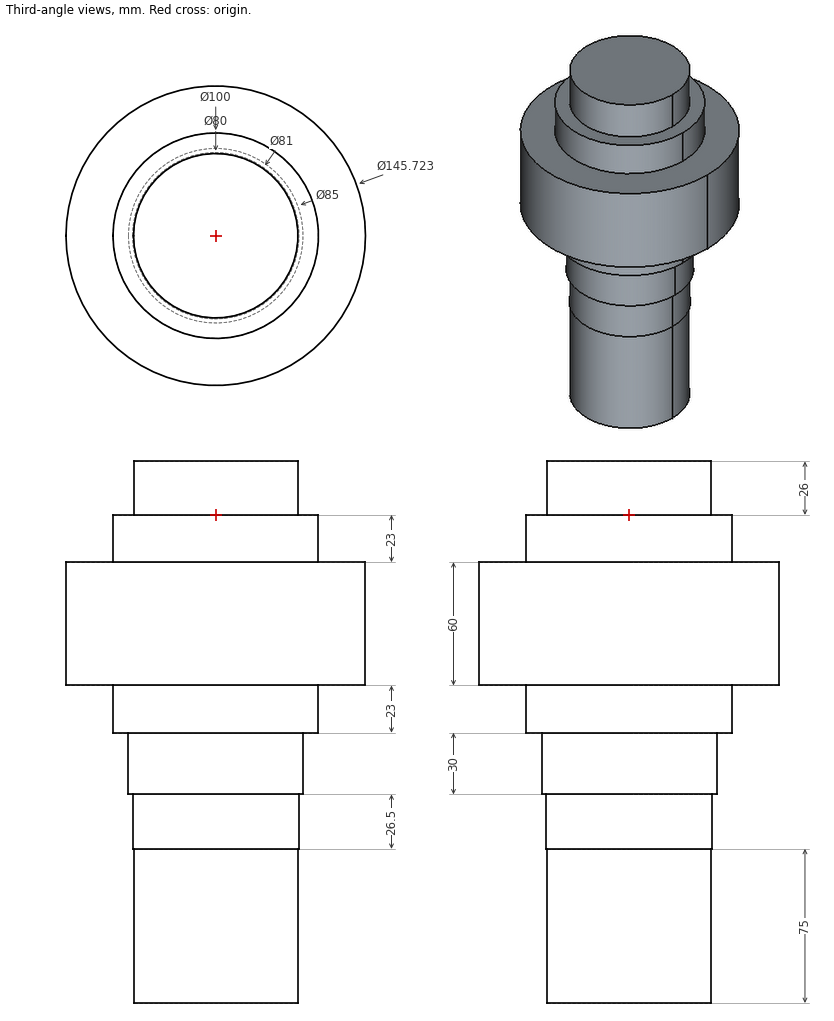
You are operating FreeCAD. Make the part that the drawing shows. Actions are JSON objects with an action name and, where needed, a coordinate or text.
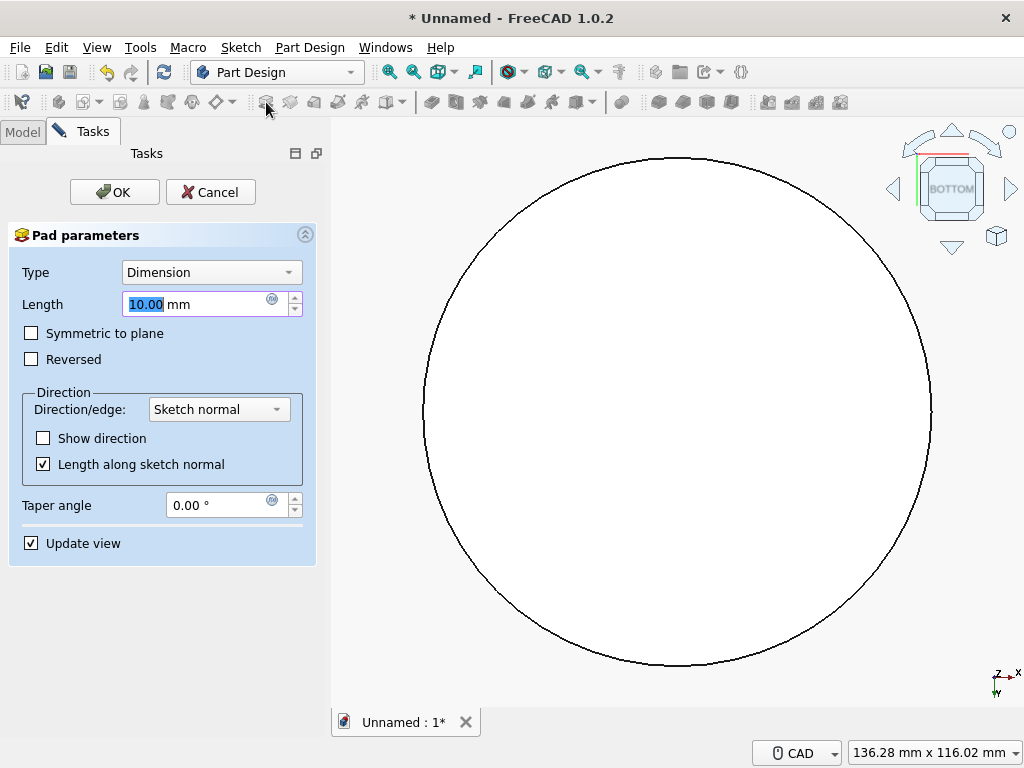
{"action": "type", "text": "23"}
{"action": "key", "text": "Tab"}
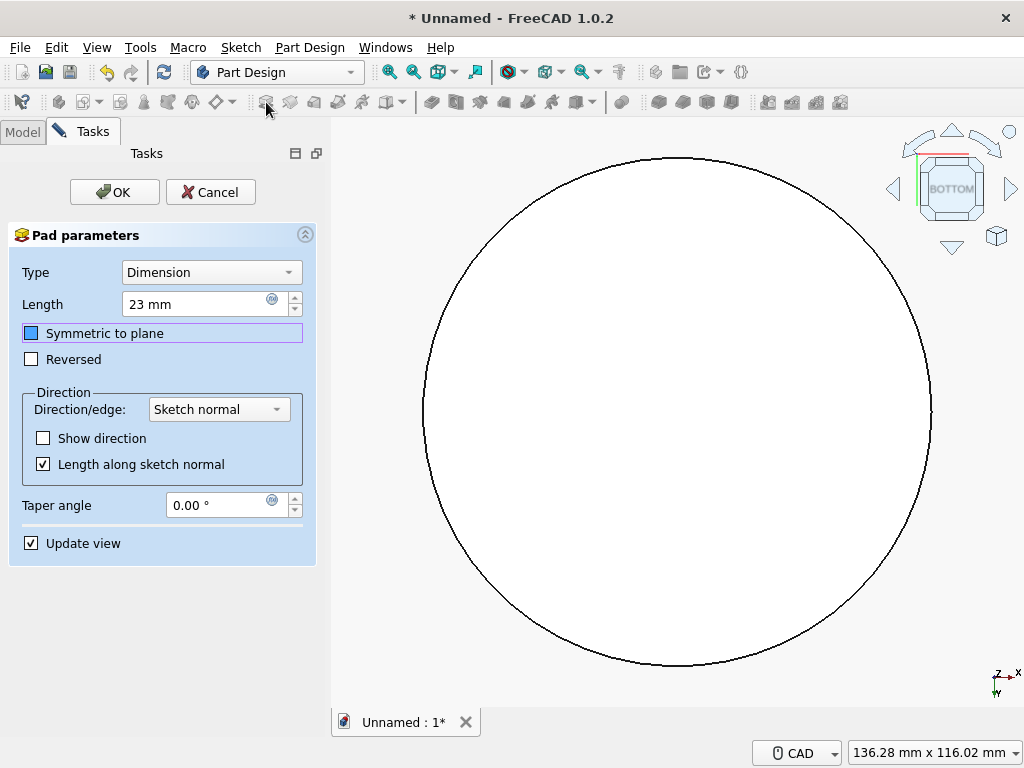
{"action": "left_click", "coordinate": [115, 192]}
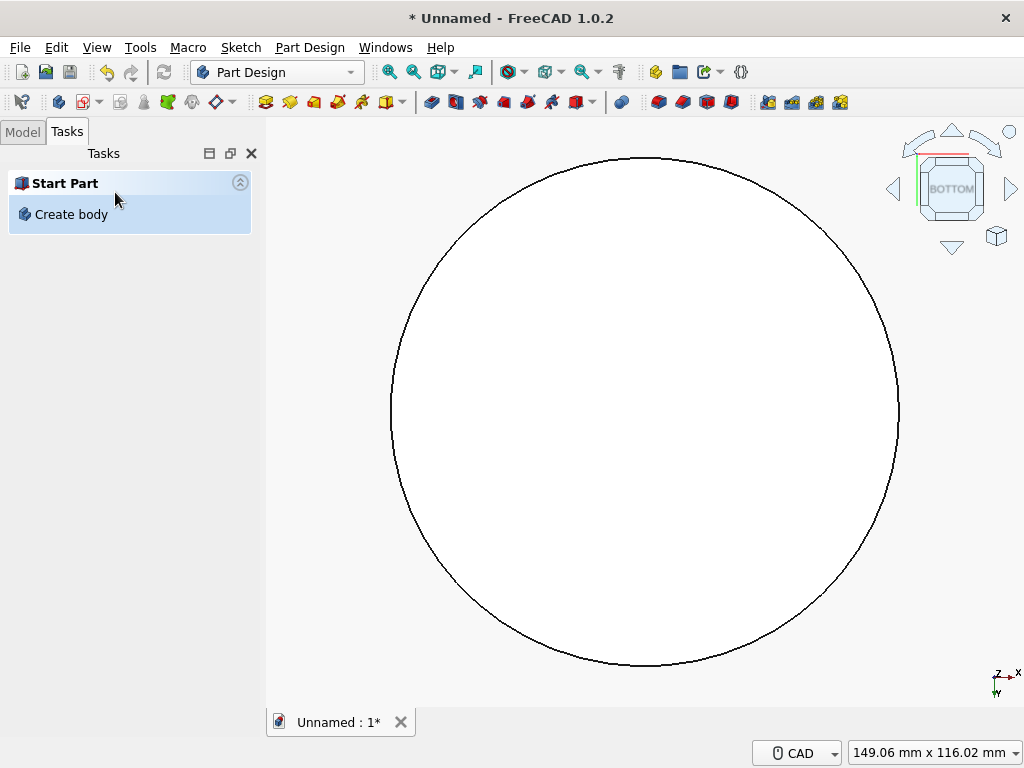
{"action": "left_click", "coordinate": [645, 411]}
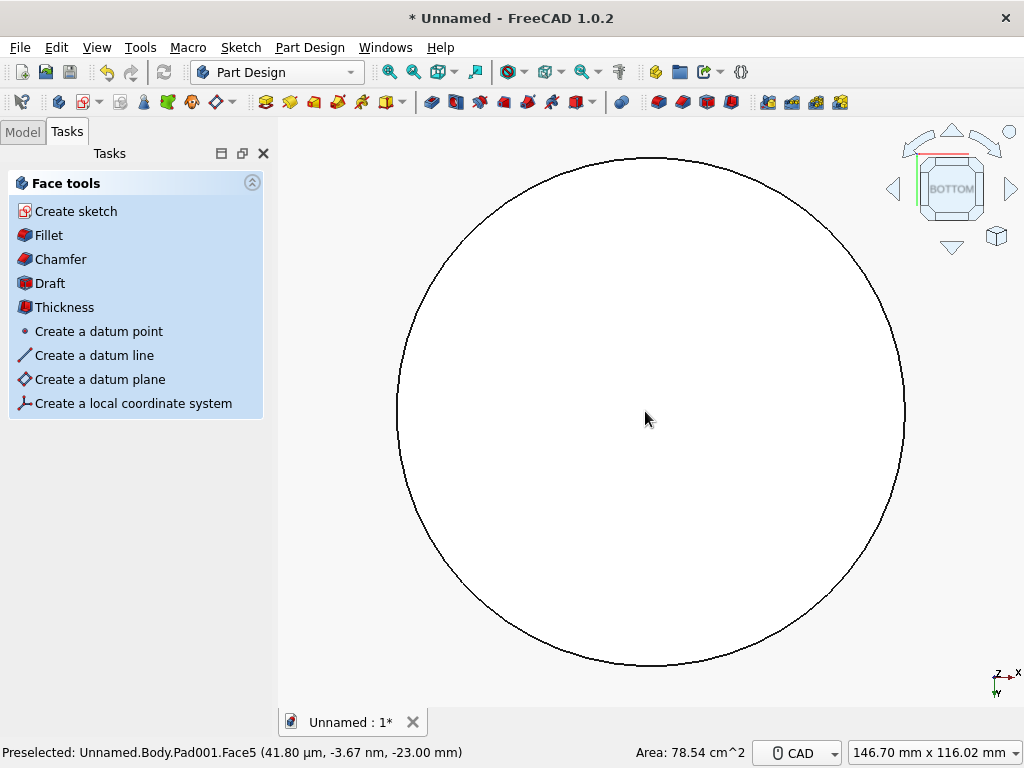
{"action": "left_click", "coordinate": [84, 102]}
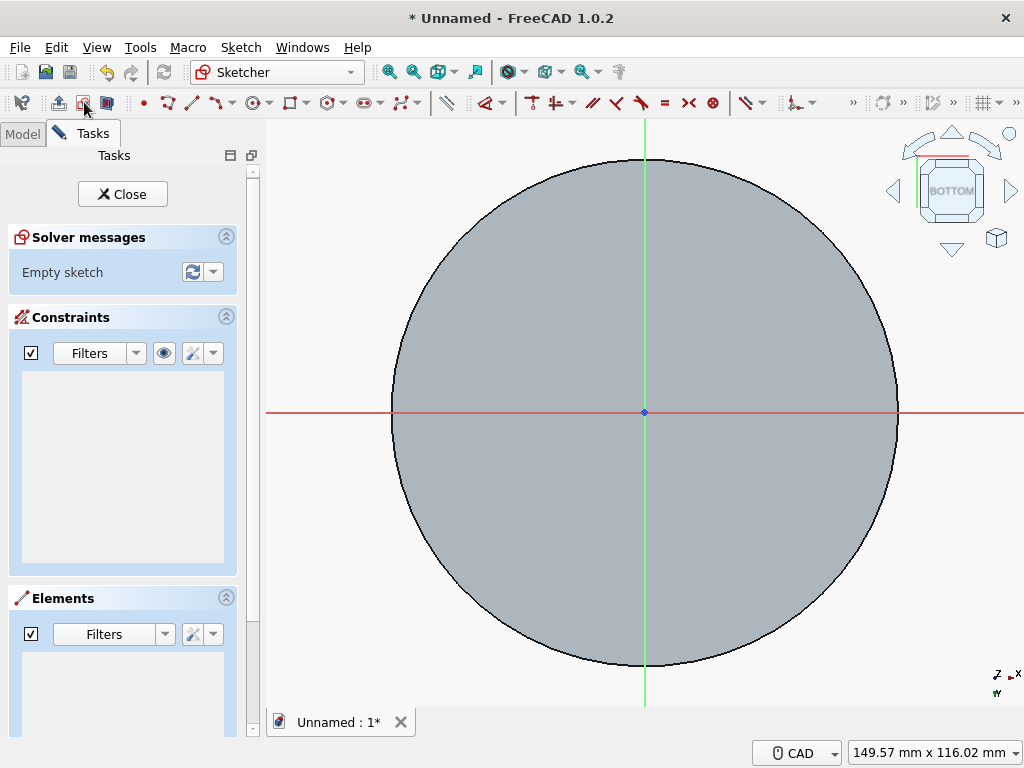
{"action": "scroll", "coordinate": [493, 413], "scroll_direction": "down", "scroll_amount": 3}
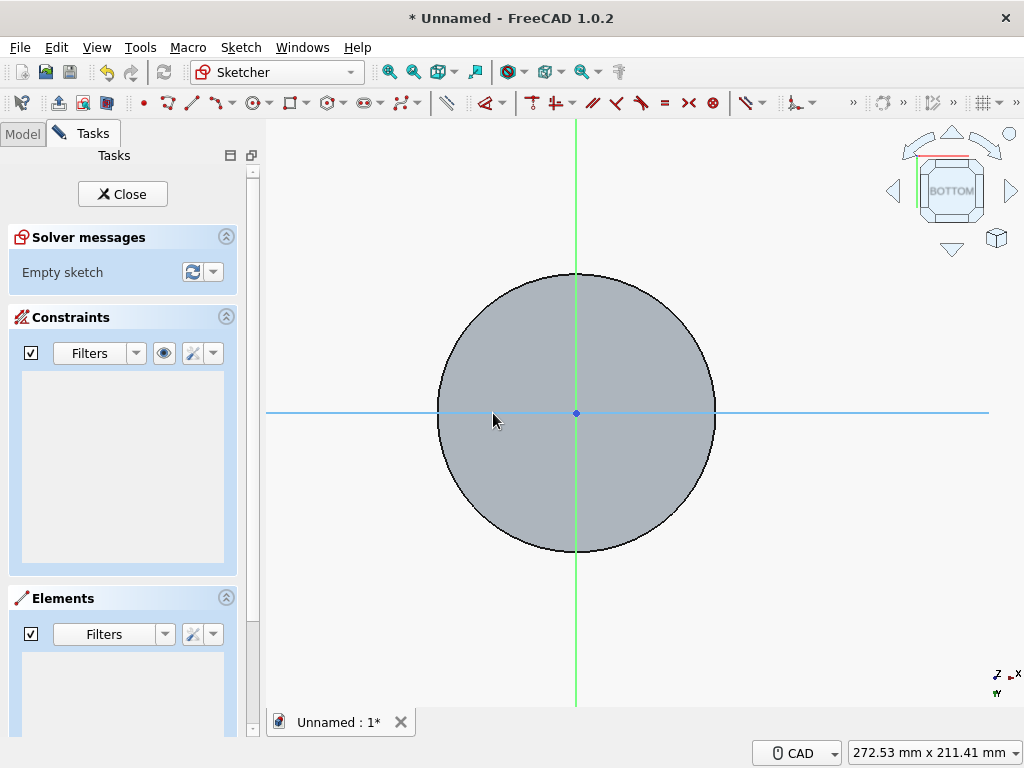
{"action": "key", "text": "g c"}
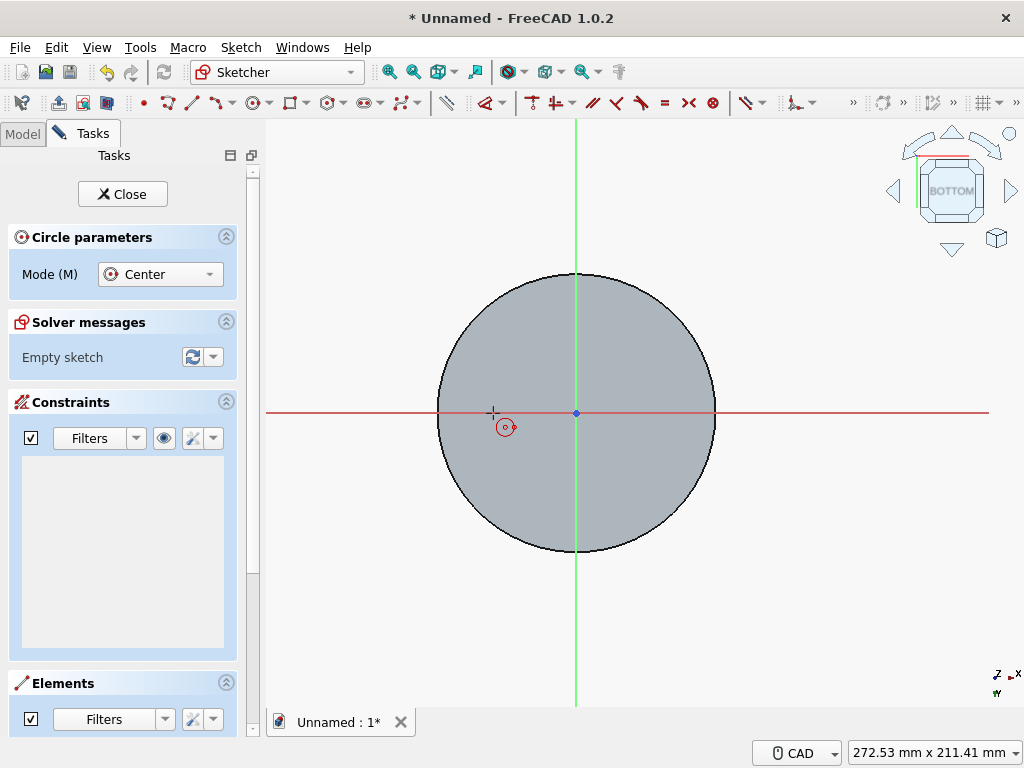
{"action": "left_click", "coordinate": [576, 413]}
{"action": "left_click", "coordinate": [720, 270]}
{"action": "key", "text": "Escape"}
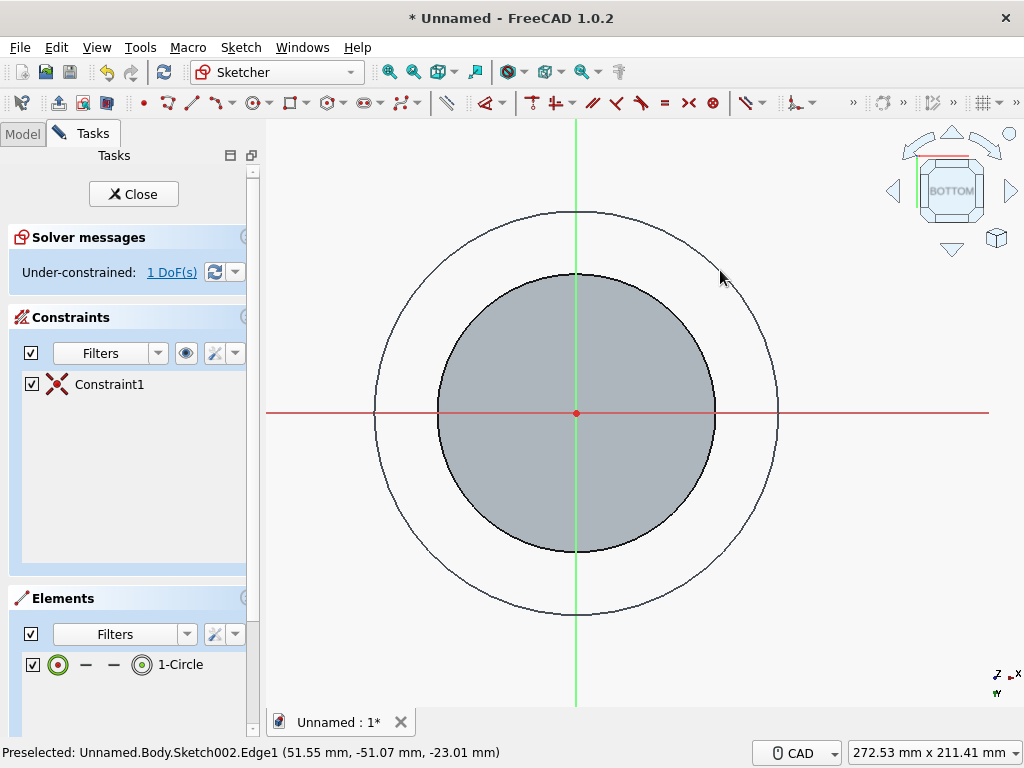
{"action": "key", "text": "d"}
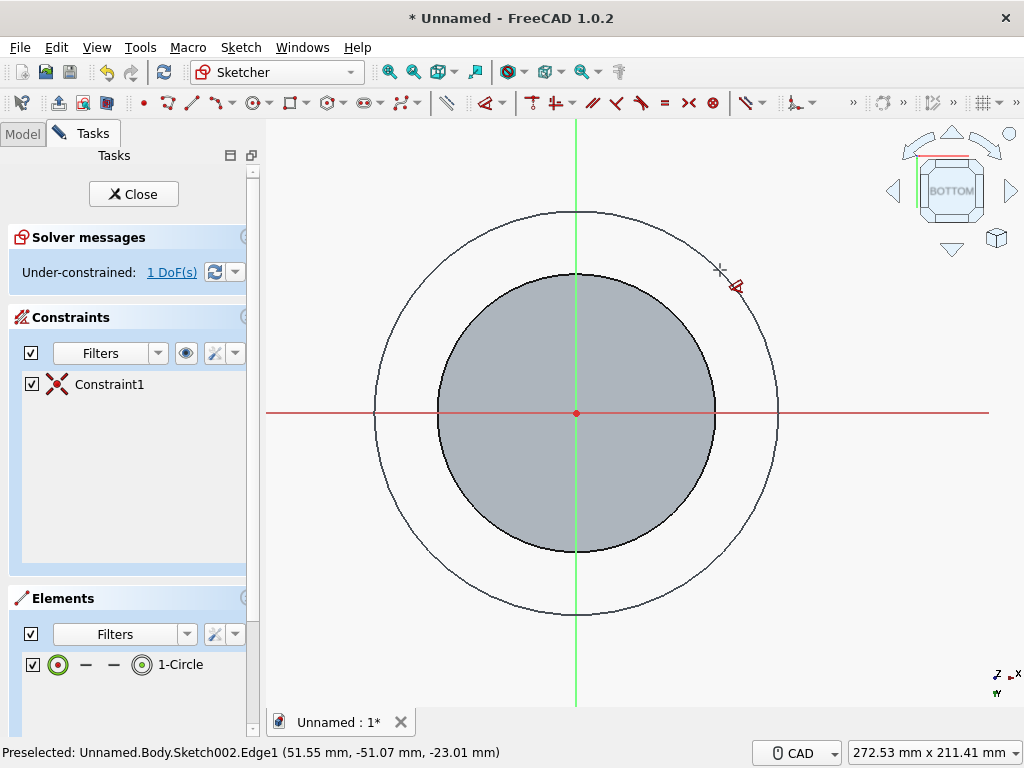
{"action": "left_click", "coordinate": [719, 270]}
{"action": "left_click", "coordinate": [742, 247]}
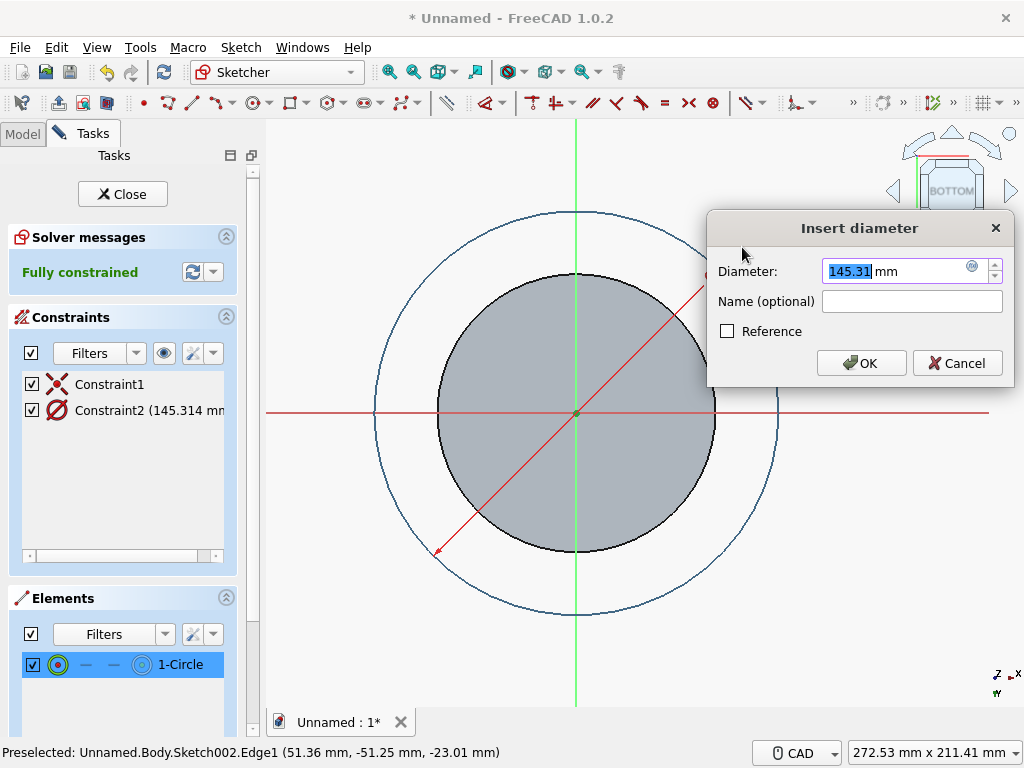
{"action": "type", "text": "145.723"}
{"action": "key", "text": "Return"}
{"action": "key", "text": "Escape"}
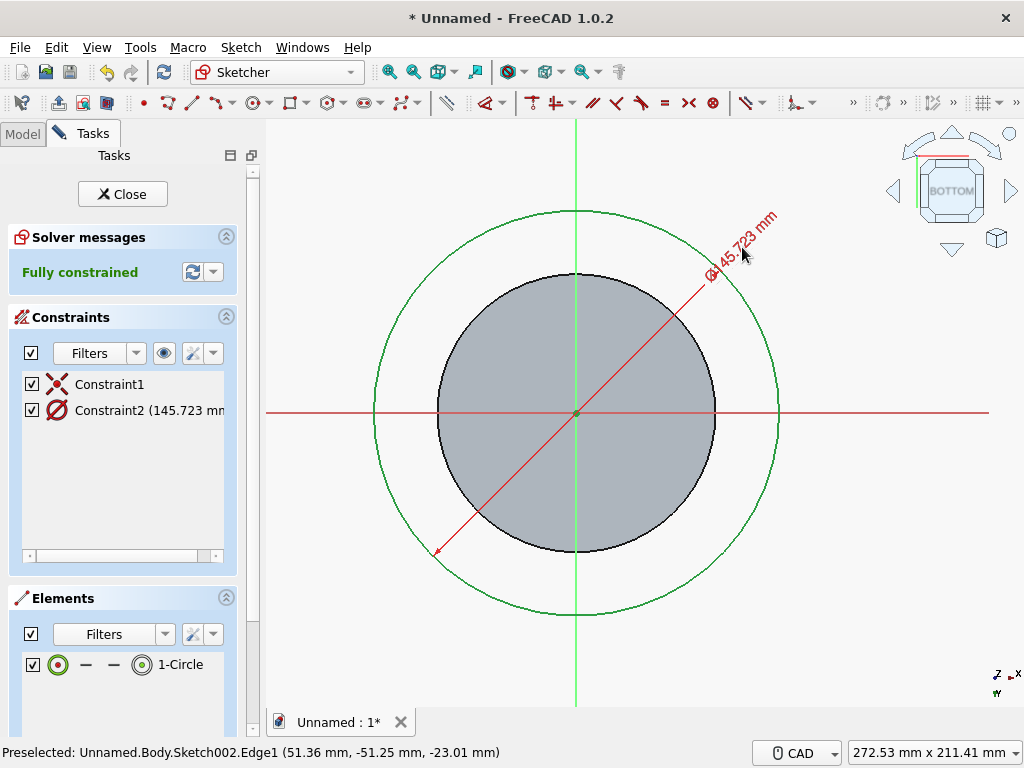
{"action": "left_click", "coordinate": [123, 194]}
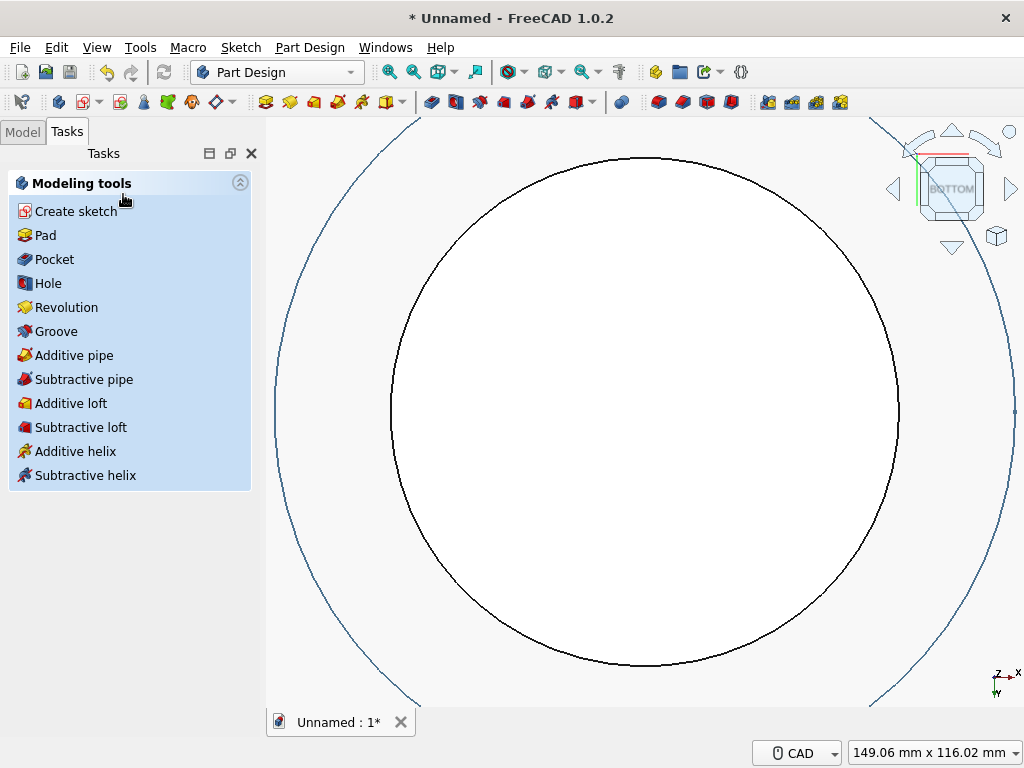
{"action": "left_click", "coordinate": [266, 102]}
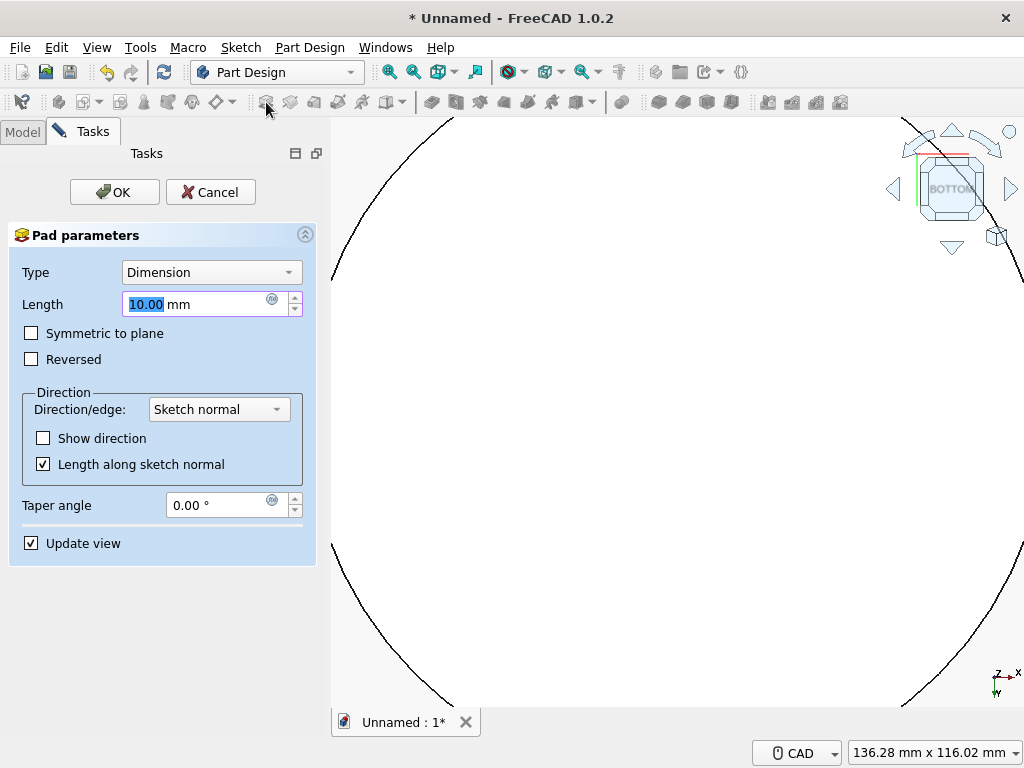
{"action": "type", "text": "60"}
{"action": "key", "text": "Tab"}